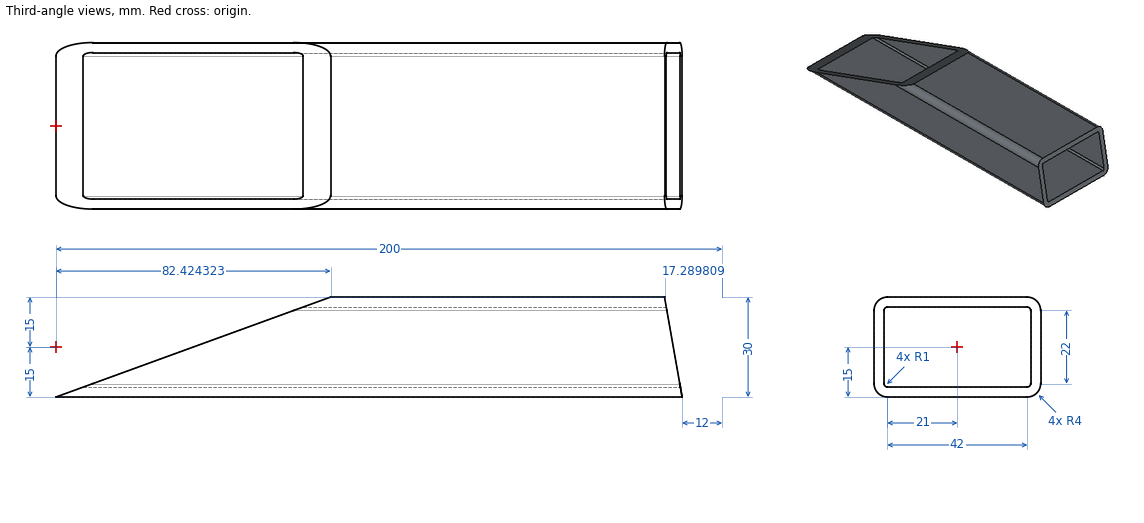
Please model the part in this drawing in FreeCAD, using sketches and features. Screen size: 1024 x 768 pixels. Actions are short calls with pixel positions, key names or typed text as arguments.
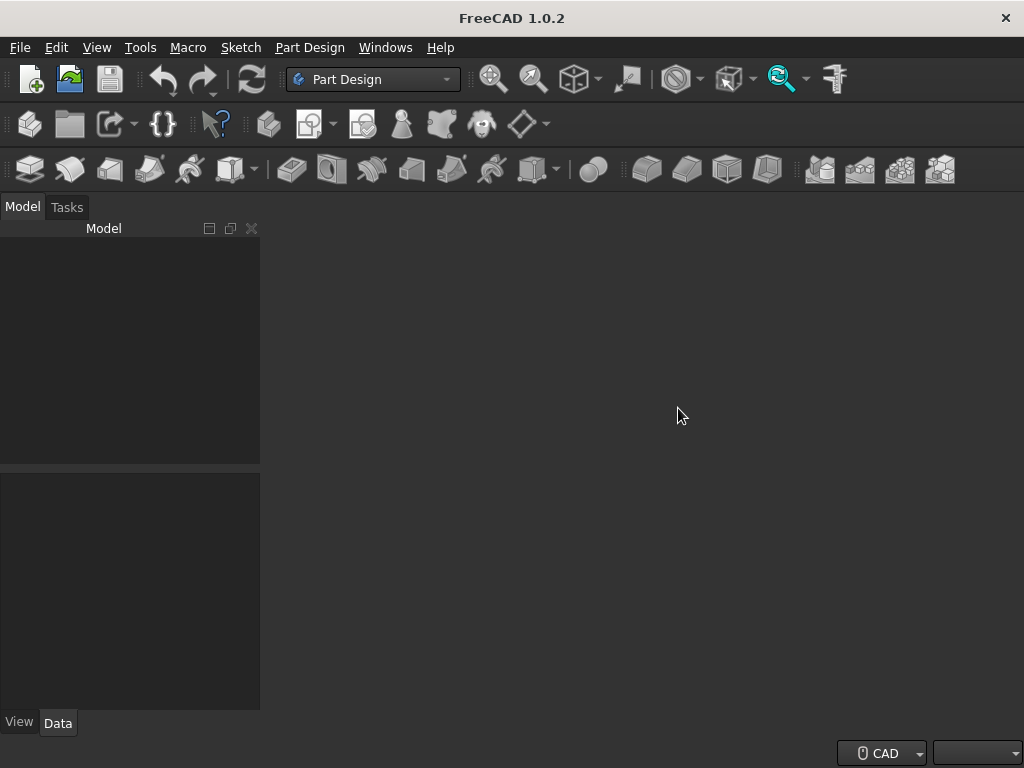
click(30, 80)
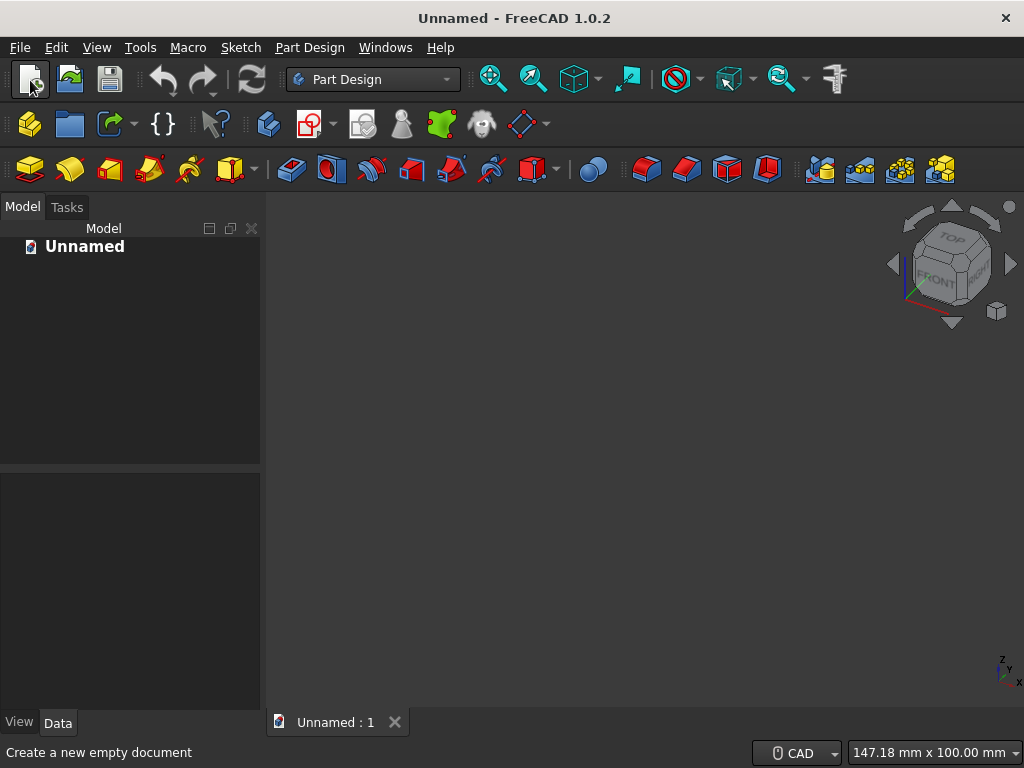
click(310, 124)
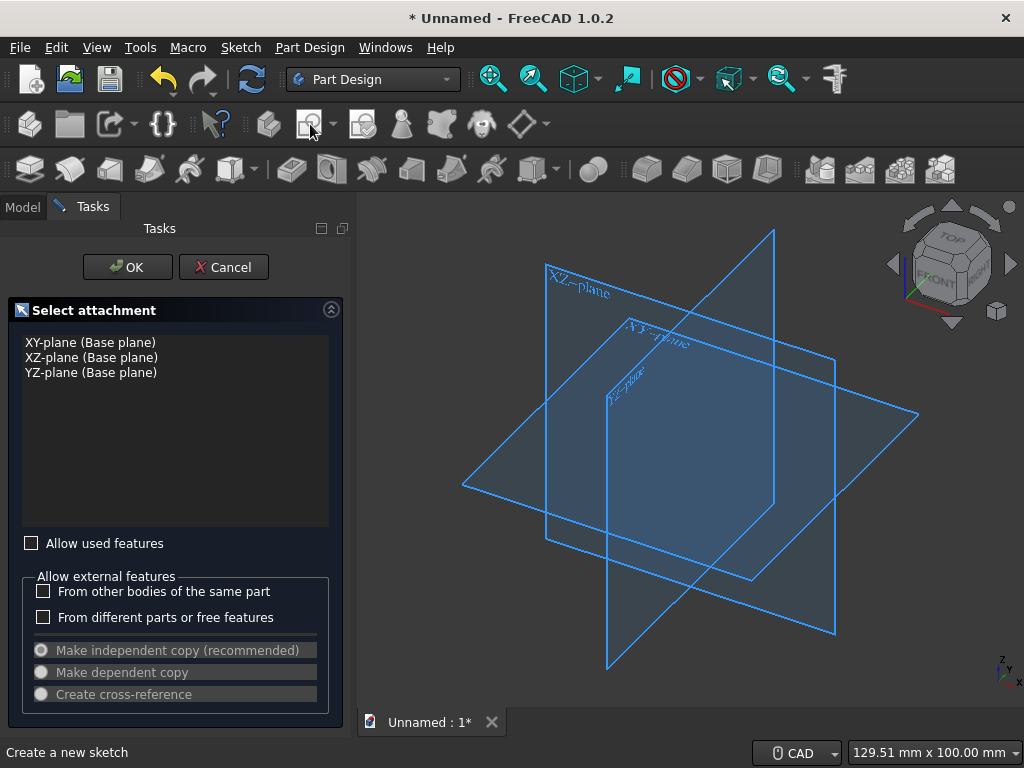
click(82, 372)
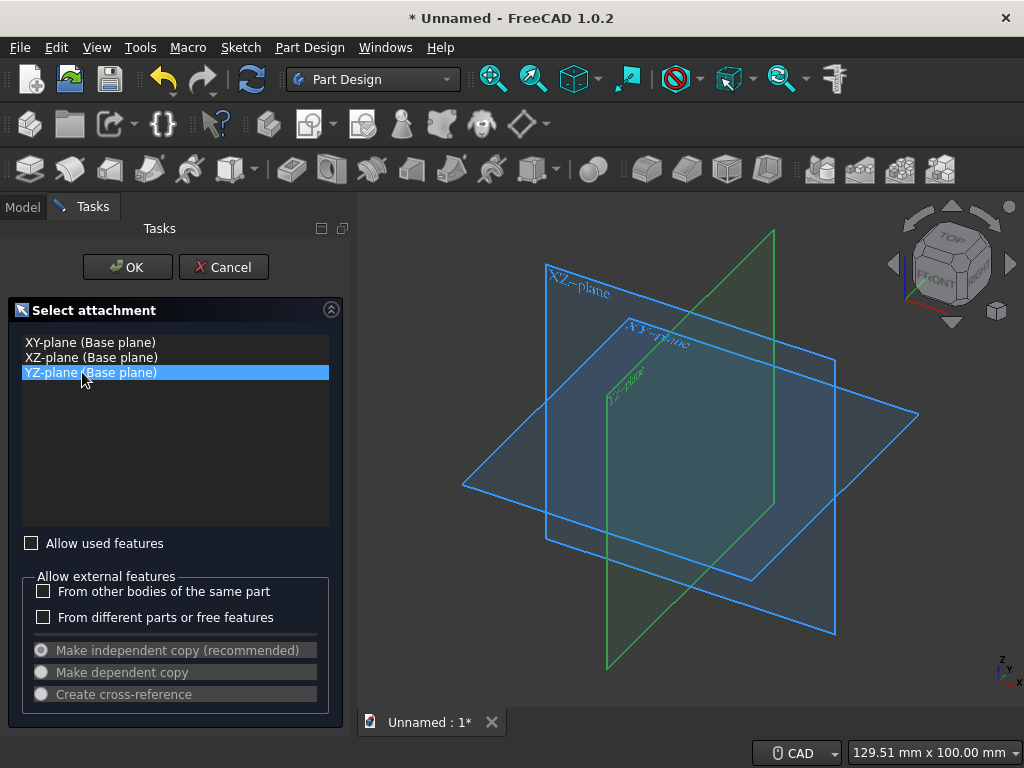
click(128, 267)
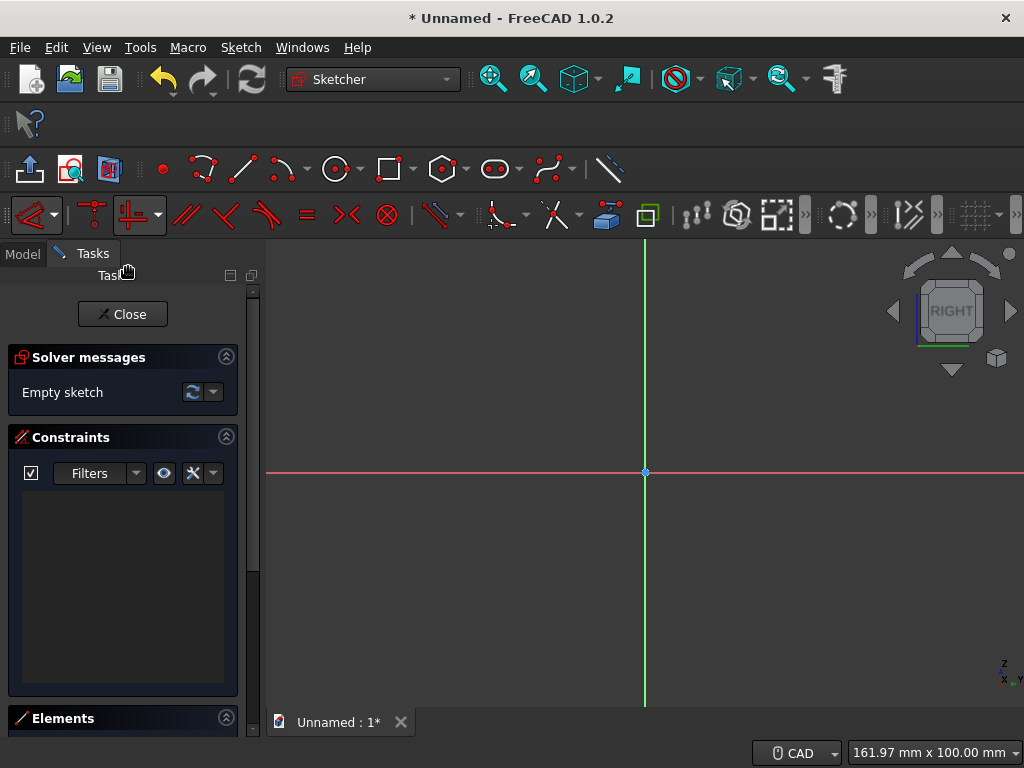
scroll(728, 473, up, 3)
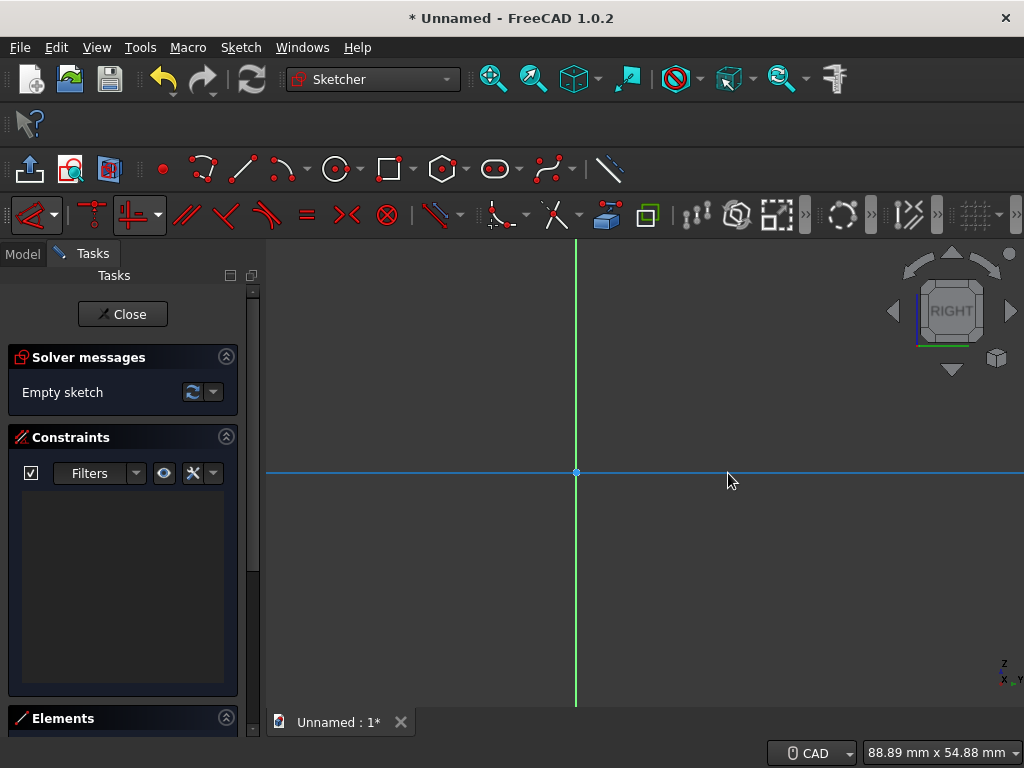
click(244, 170)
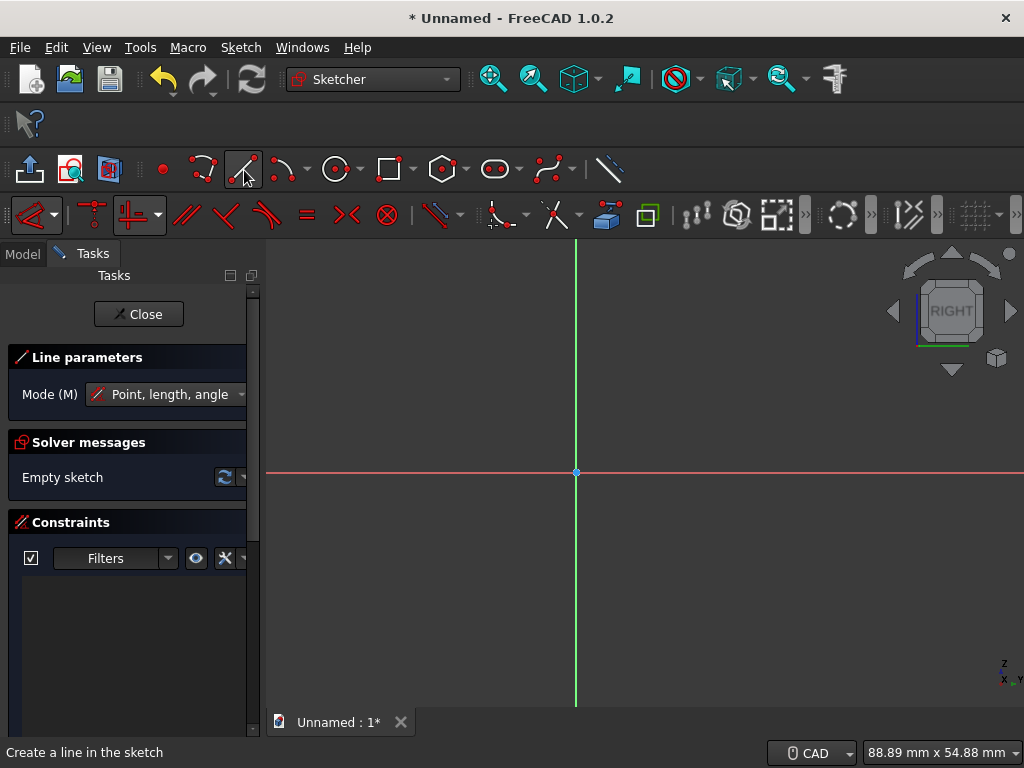
click(397, 601)
click(755, 601)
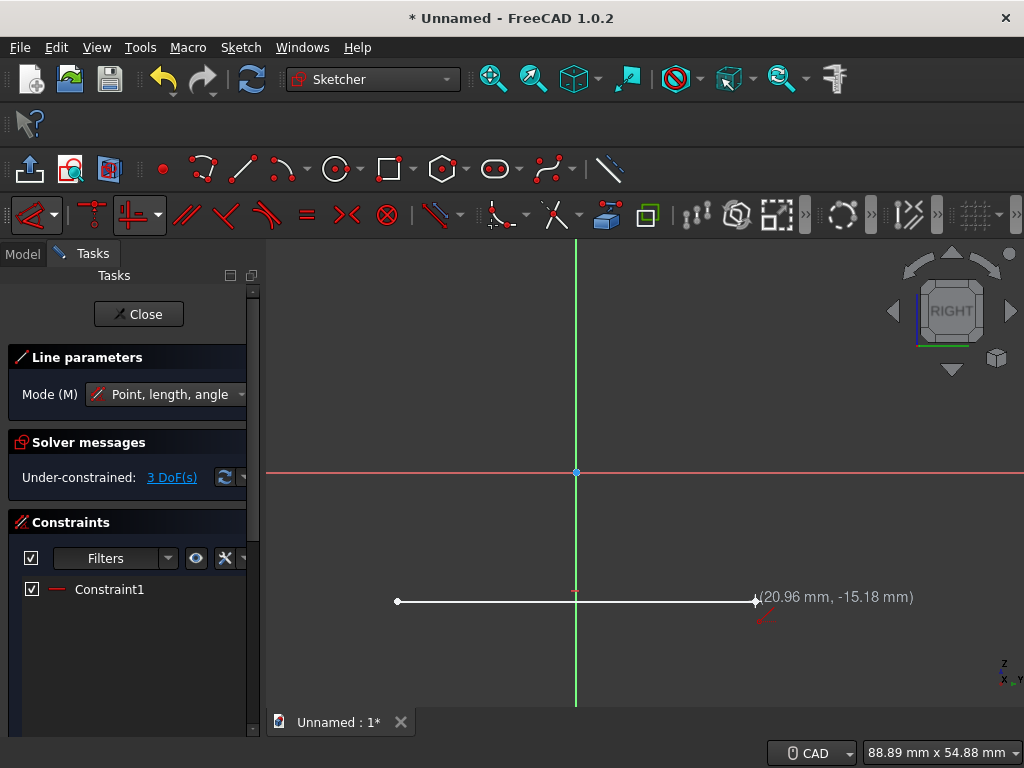
click(789, 566)
click(789, 379)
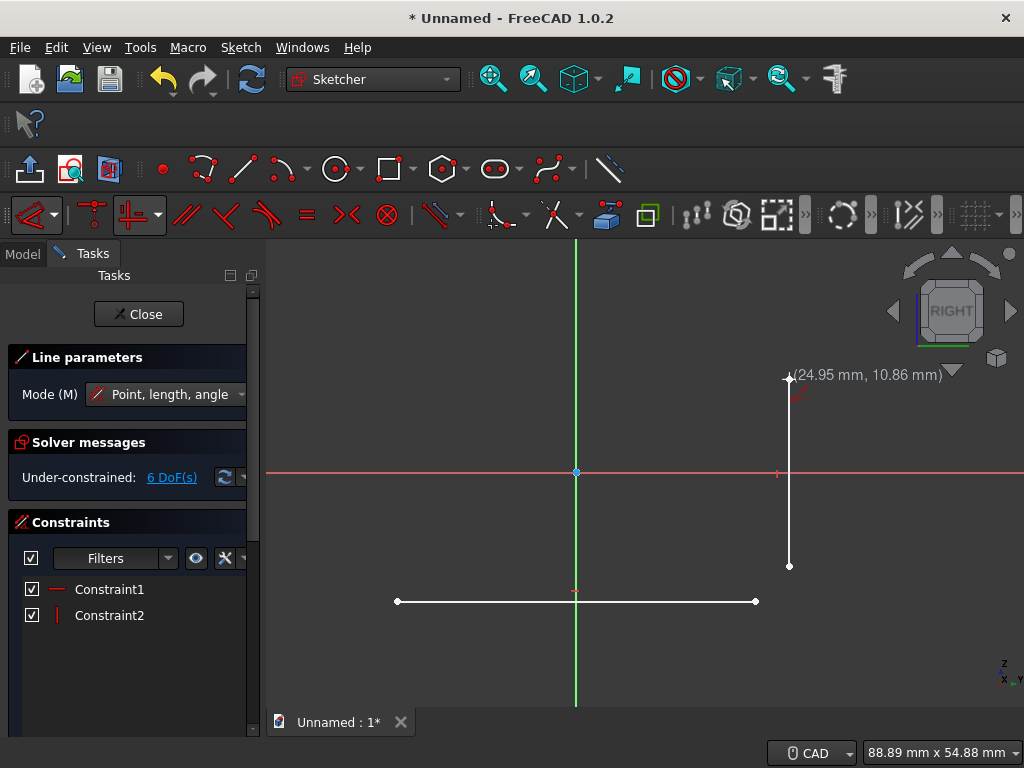
click(755, 345)
click(397, 345)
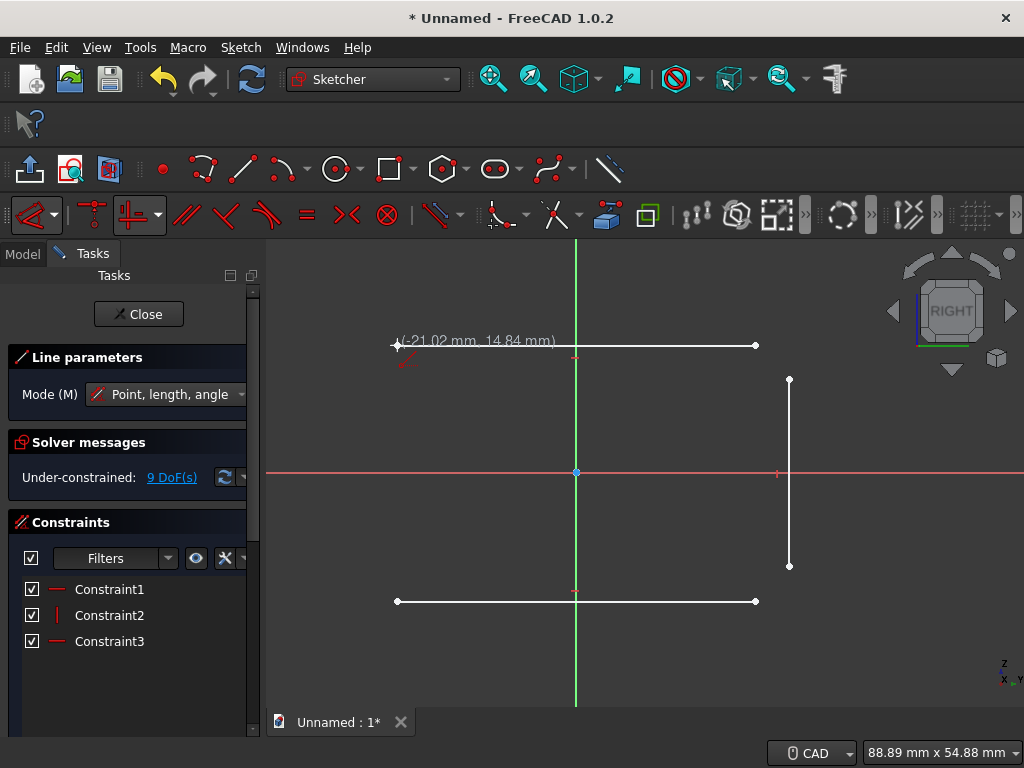
click(363, 379)
click(363, 566)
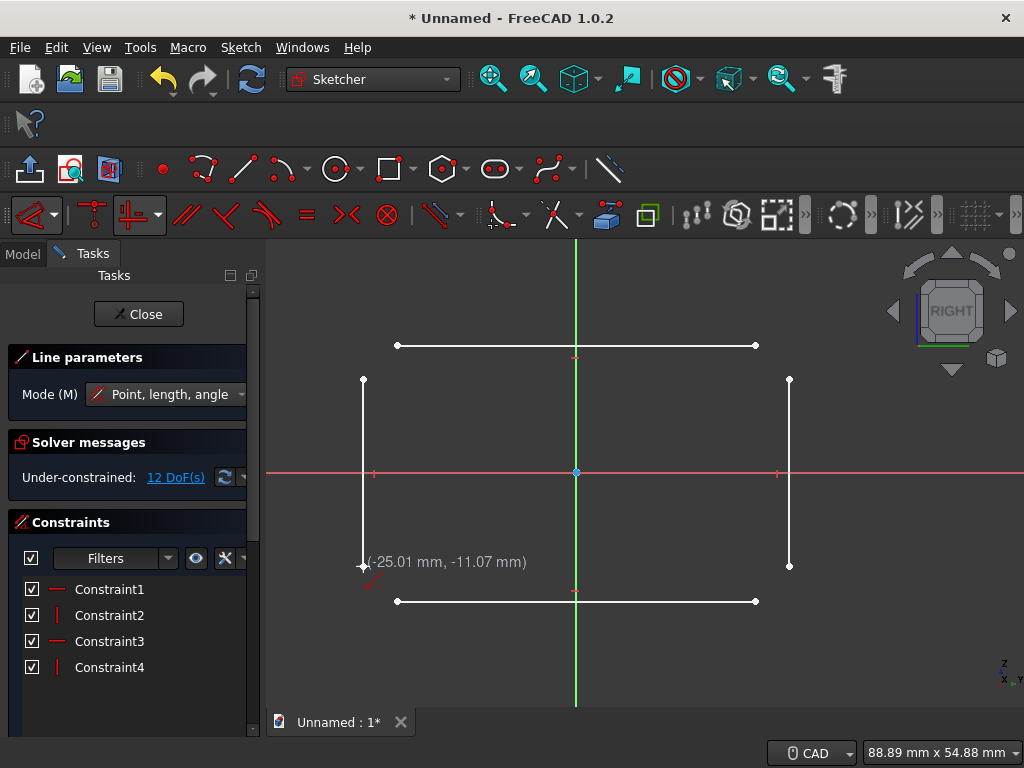
click(310, 170)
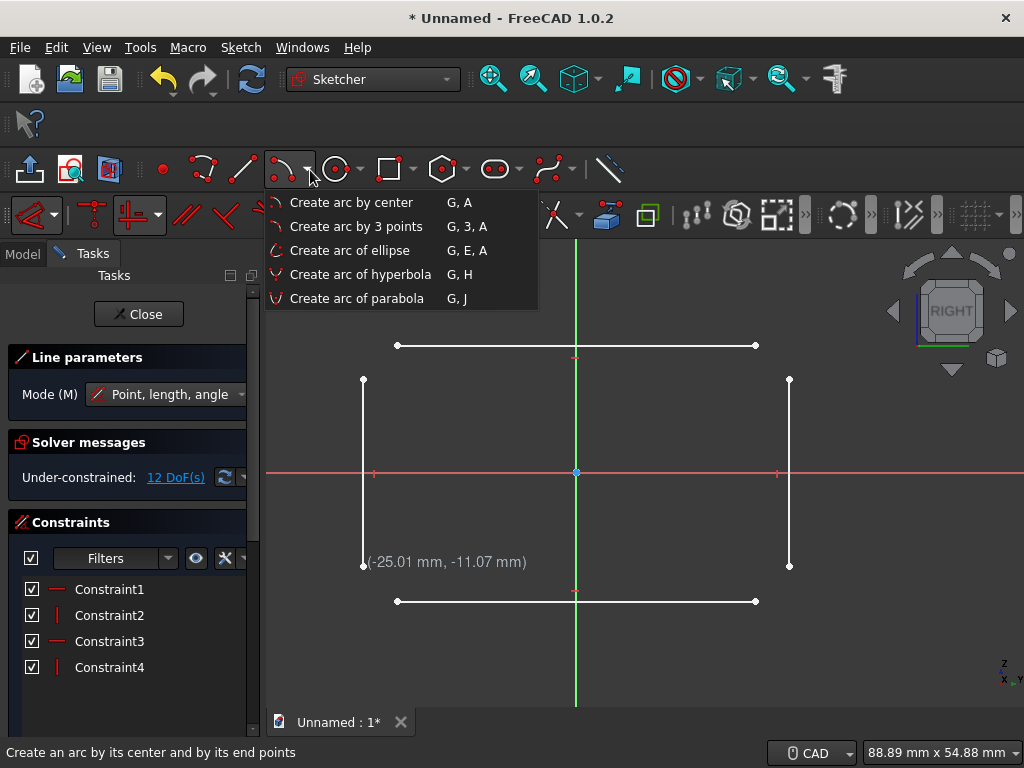
click(402, 226)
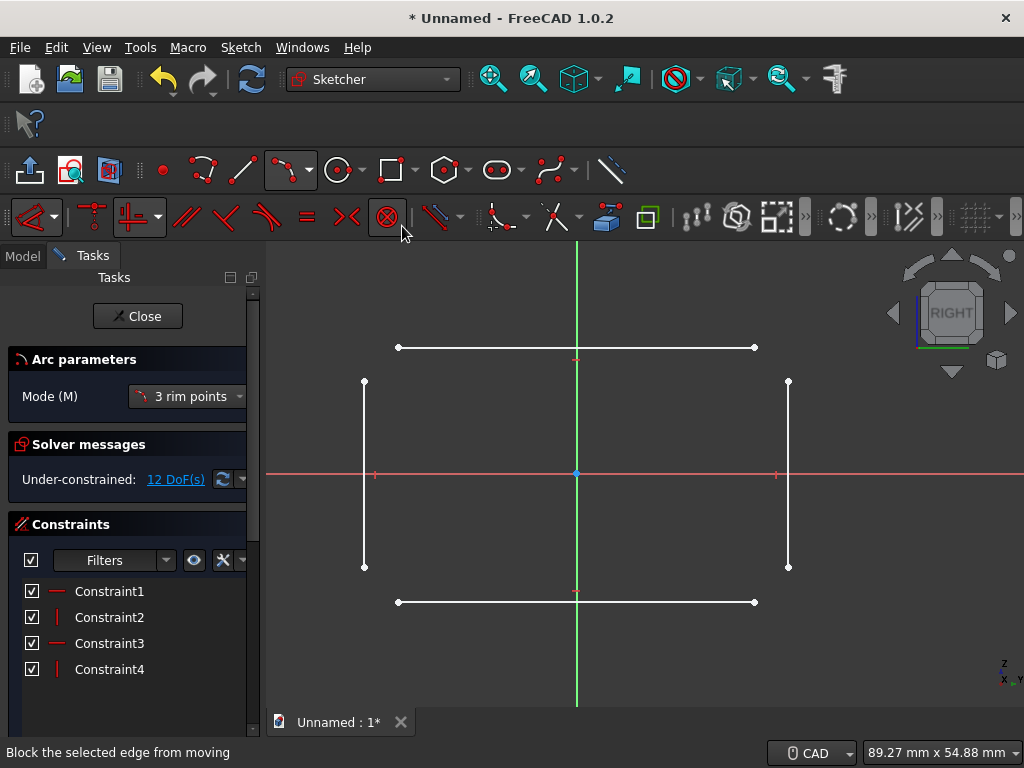
click(755, 602)
click(788, 568)